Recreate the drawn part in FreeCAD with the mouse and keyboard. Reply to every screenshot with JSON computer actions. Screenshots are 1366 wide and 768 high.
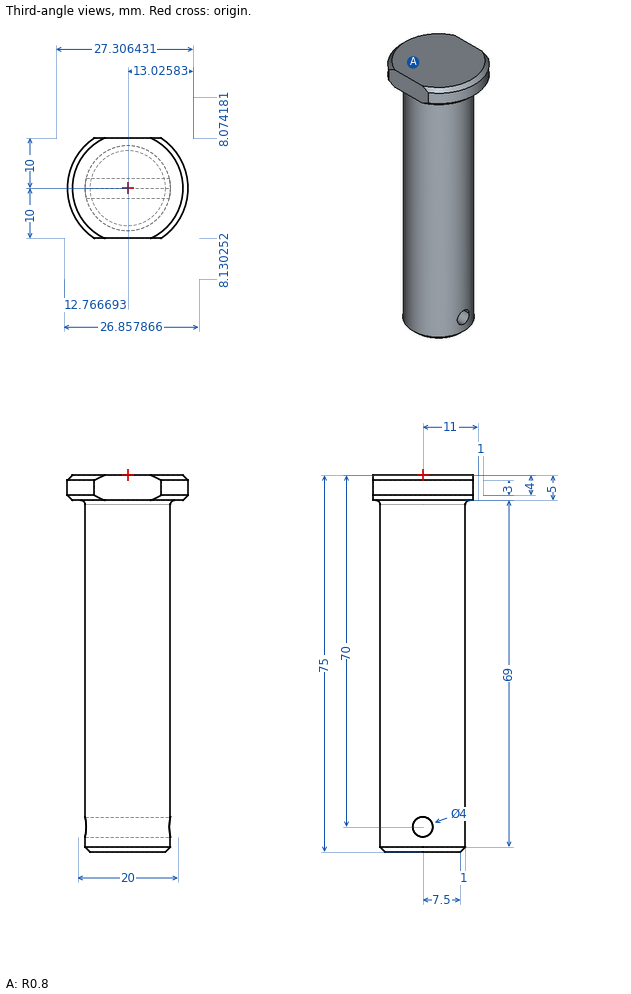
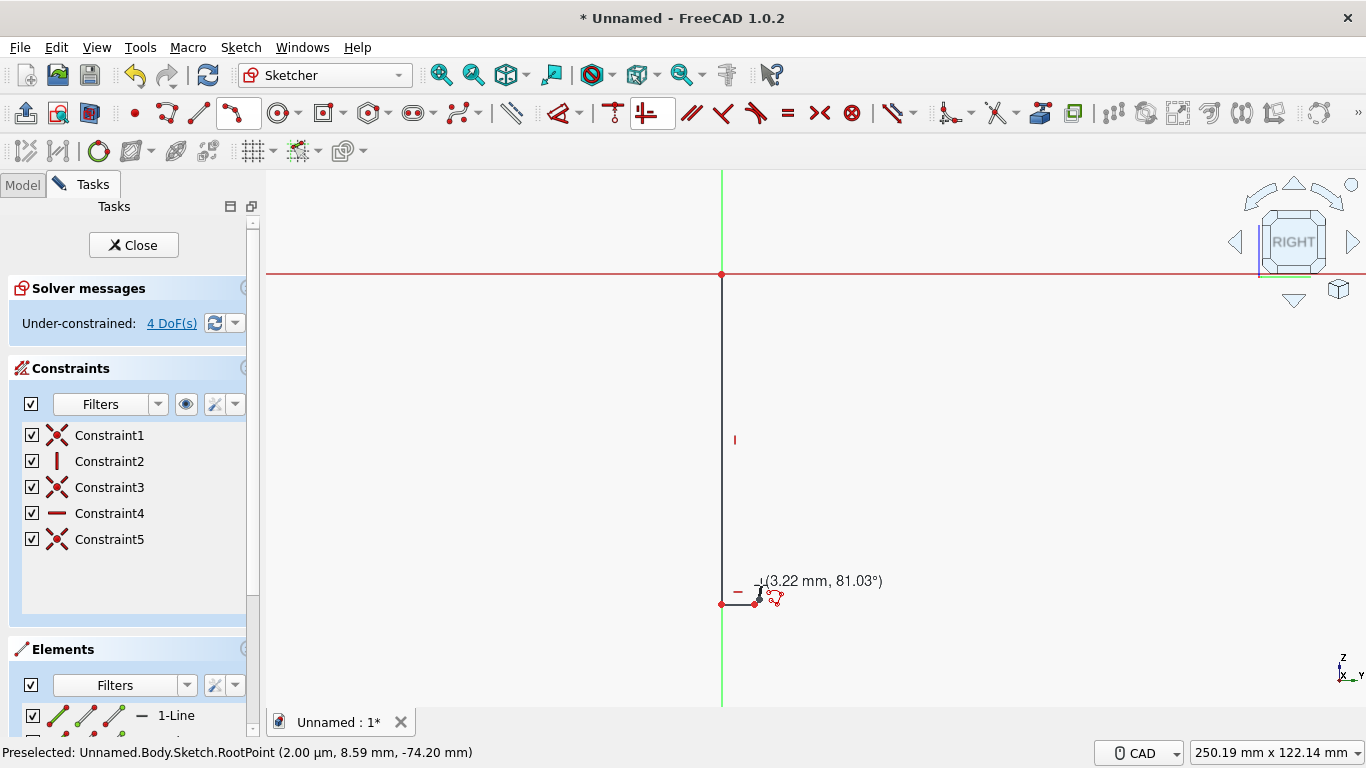
{"action": "left_click", "coordinate": [759, 296]}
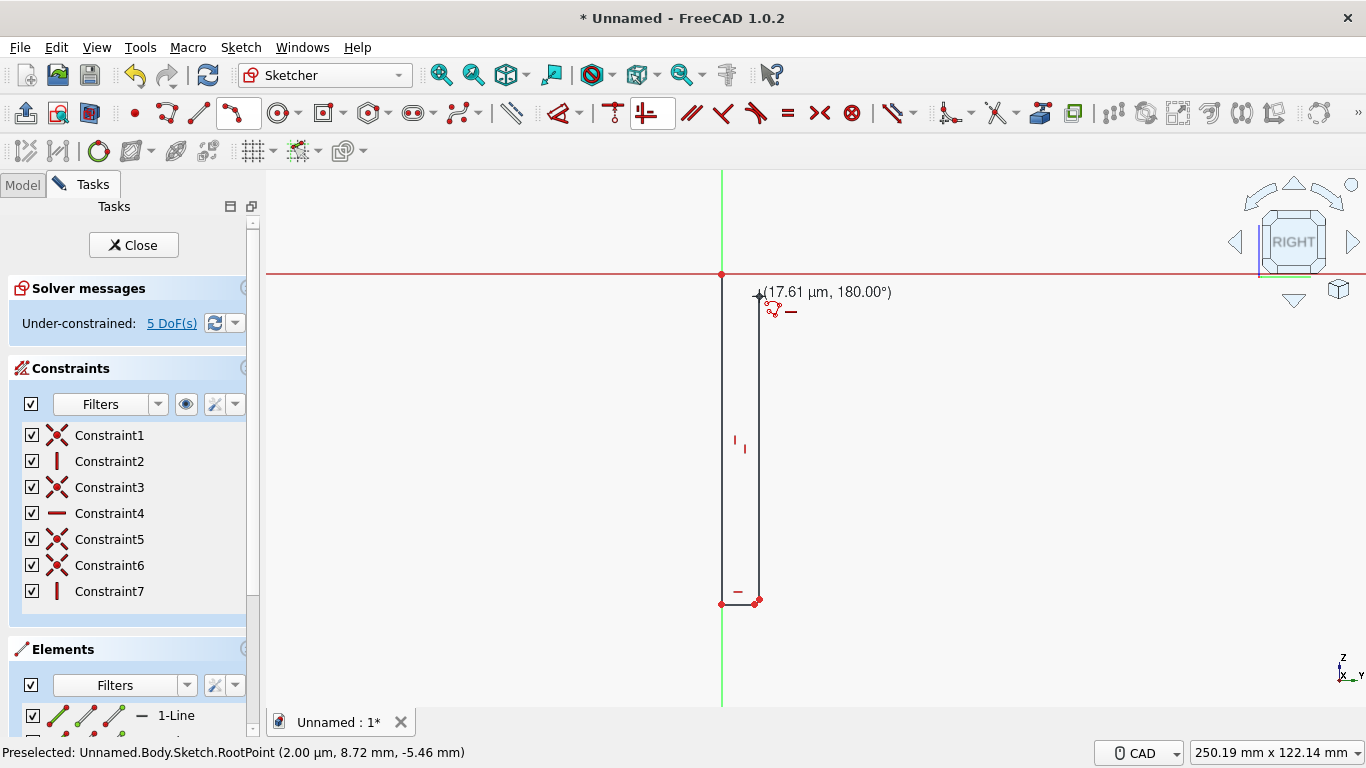
{"action": "scroll", "coordinate": [770, 296], "scroll_direction": "up", "scroll_amount": 2}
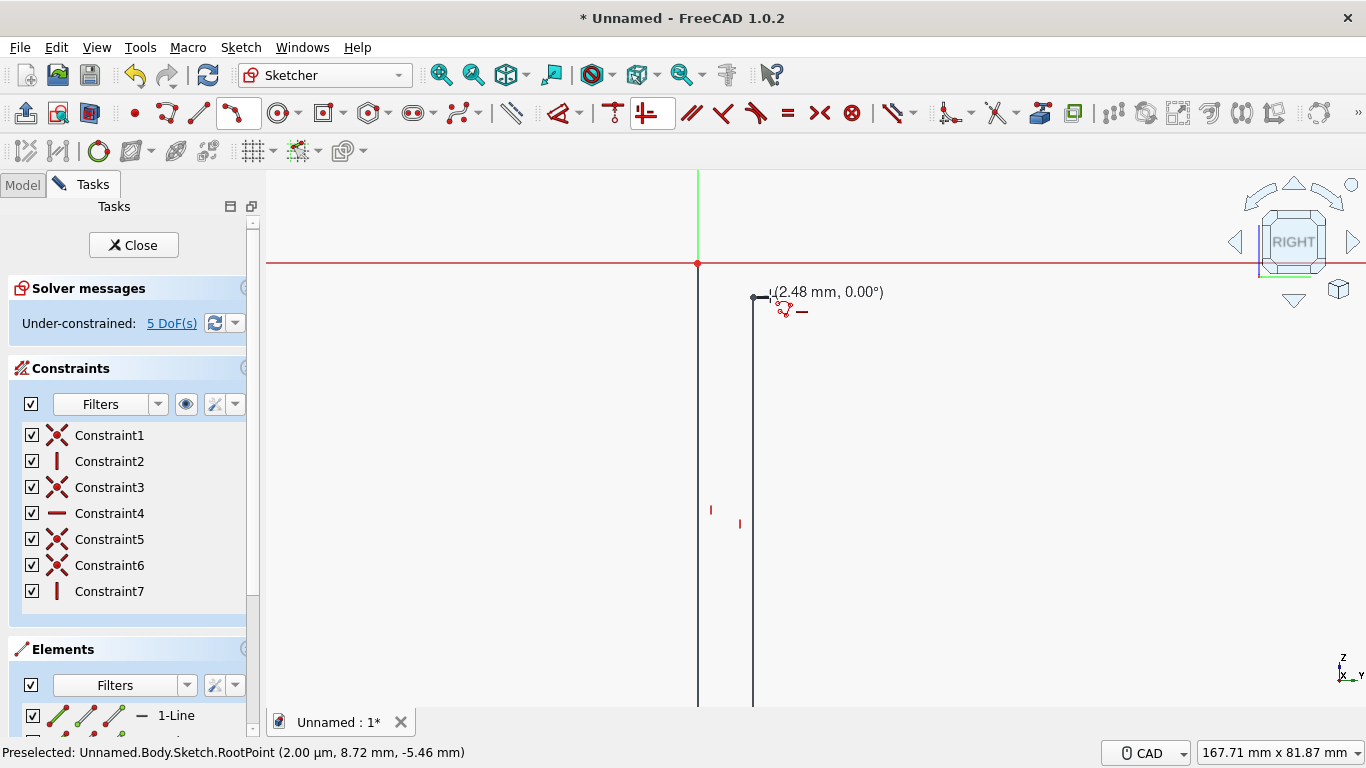
{"action": "left_click", "coordinate": [770, 296]}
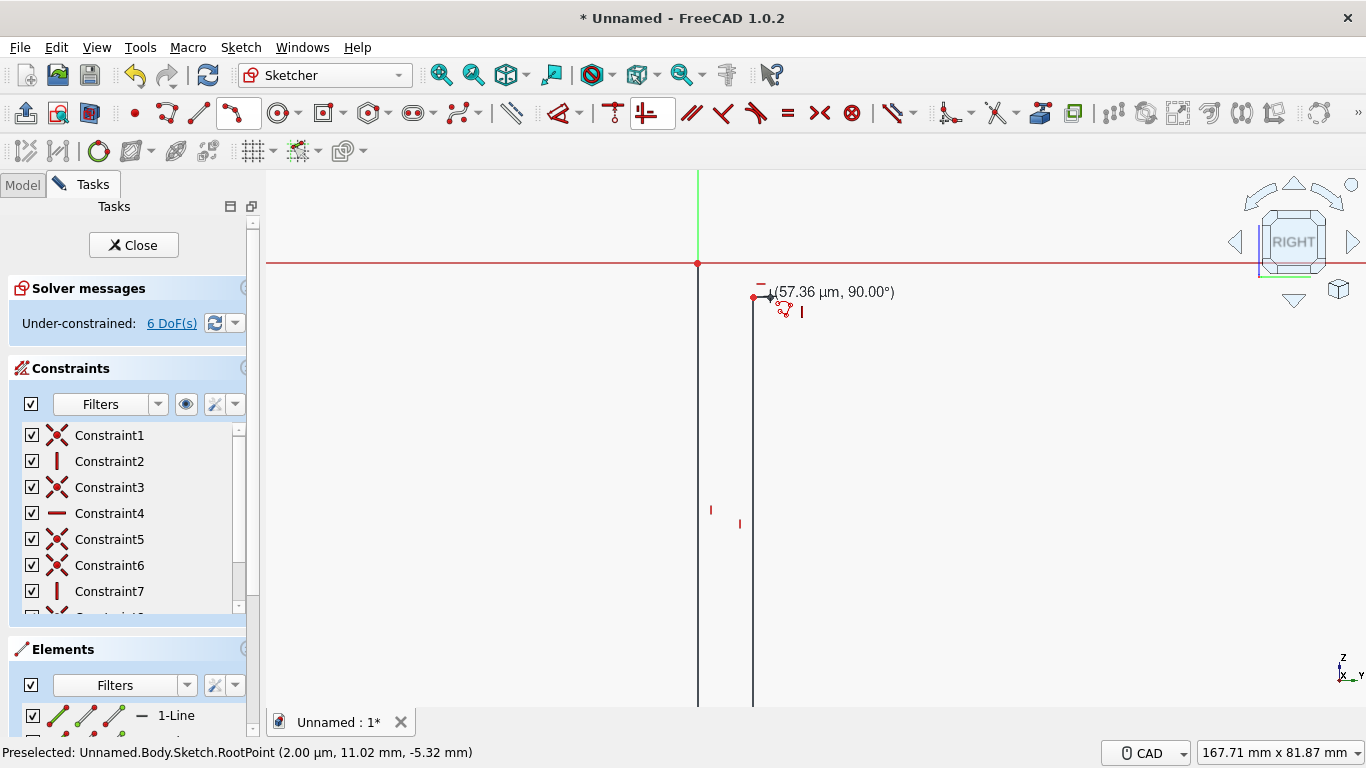
{"action": "scroll", "coordinate": [776, 289], "scroll_direction": "up", "scroll_amount": 3}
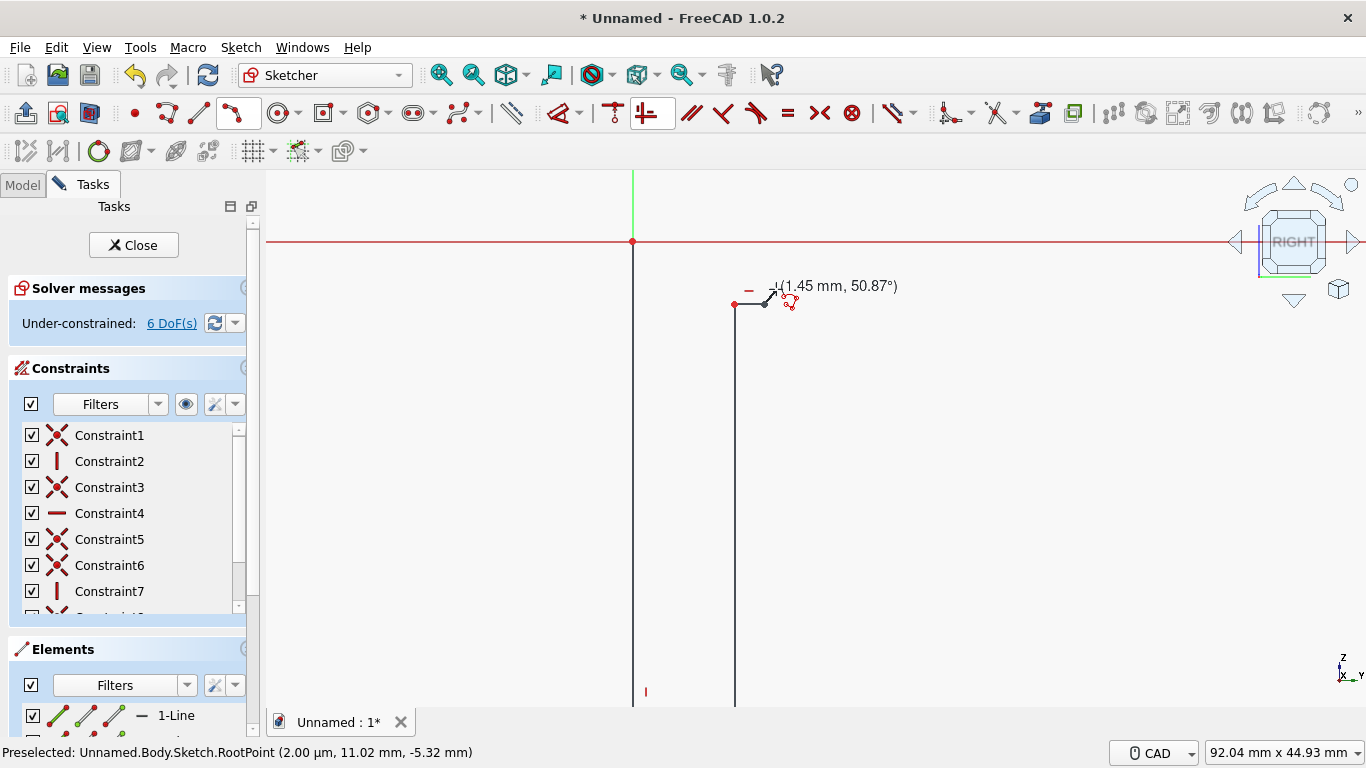
{"action": "left_click", "coordinate": [776, 289]}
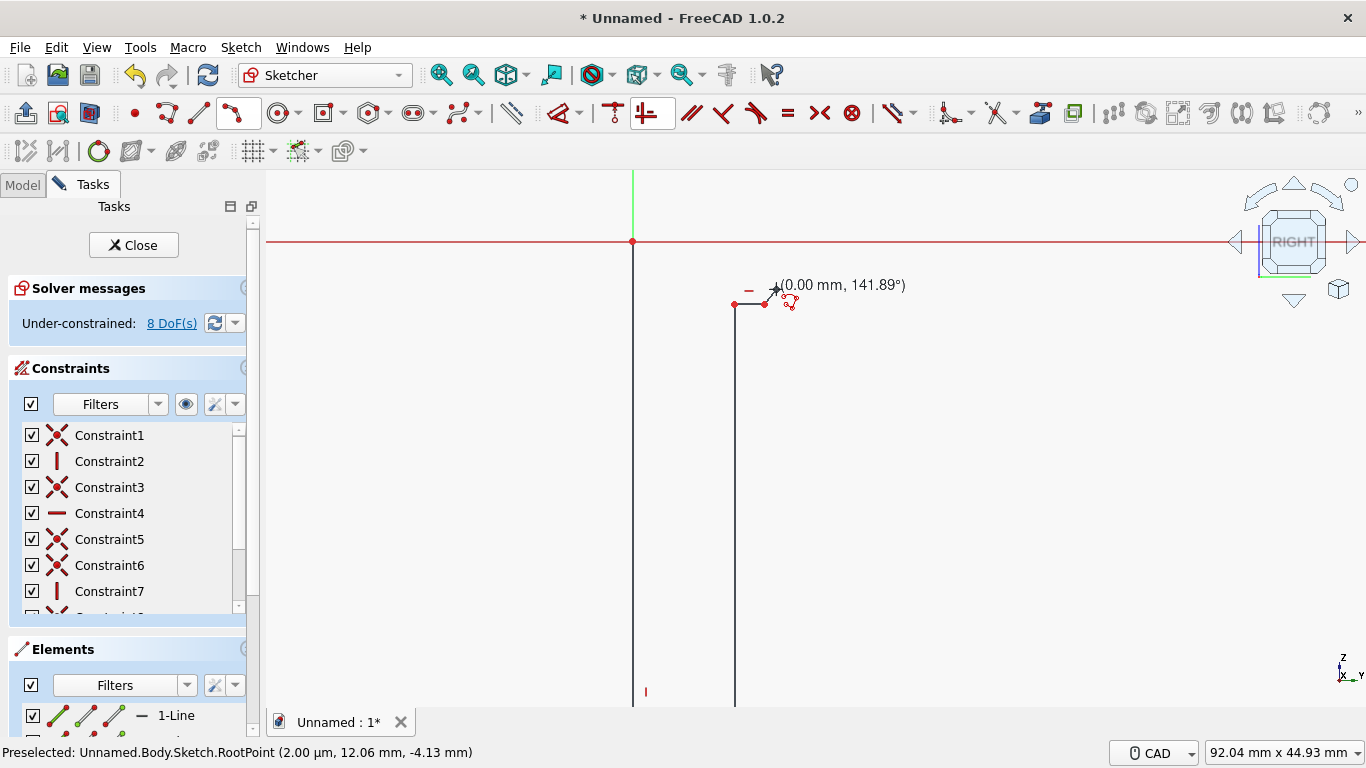
{"action": "scroll", "coordinate": [776, 254], "scroll_direction": "up", "scroll_amount": 2}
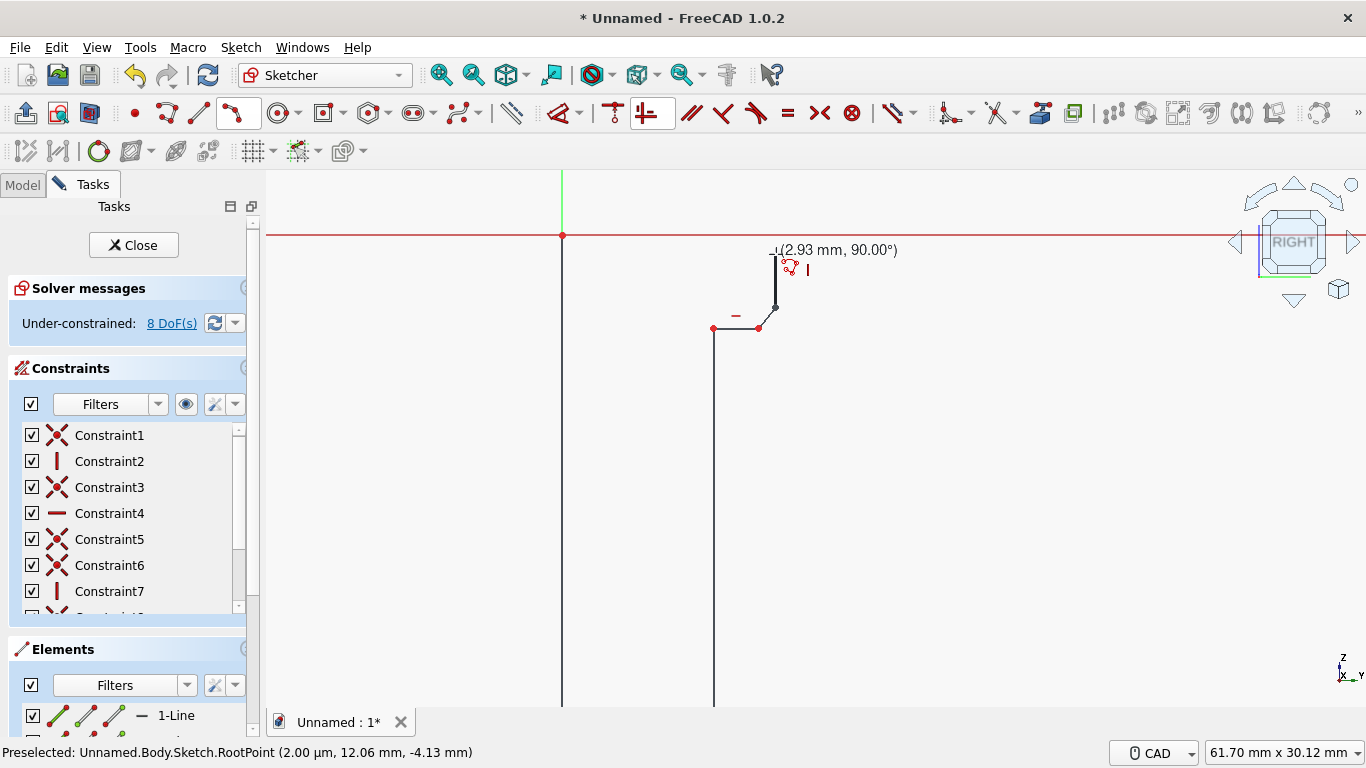
{"action": "left_click", "coordinate": [776, 253]}
{"action": "left_click", "coordinate": [758, 244]}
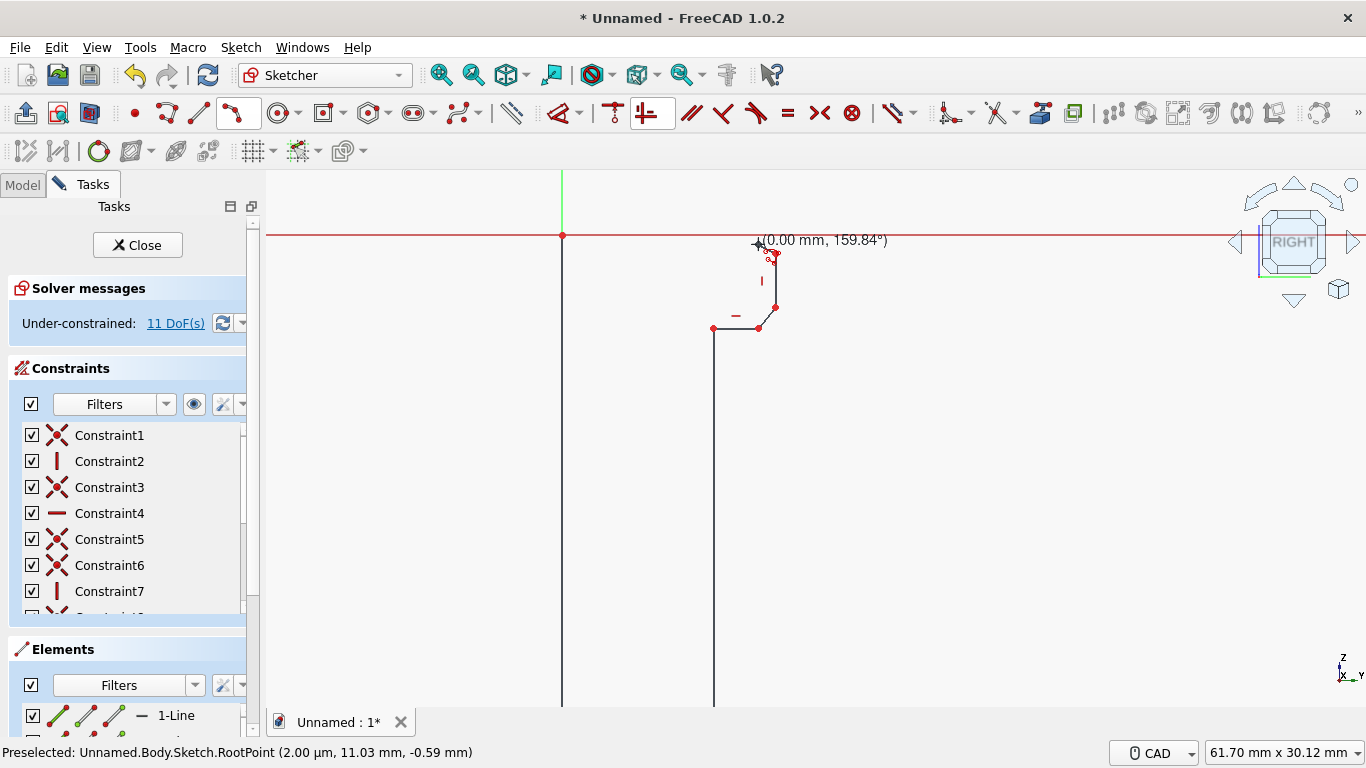
{"action": "scroll", "coordinate": [773, 286], "scroll_direction": "down", "scroll_amount": 7}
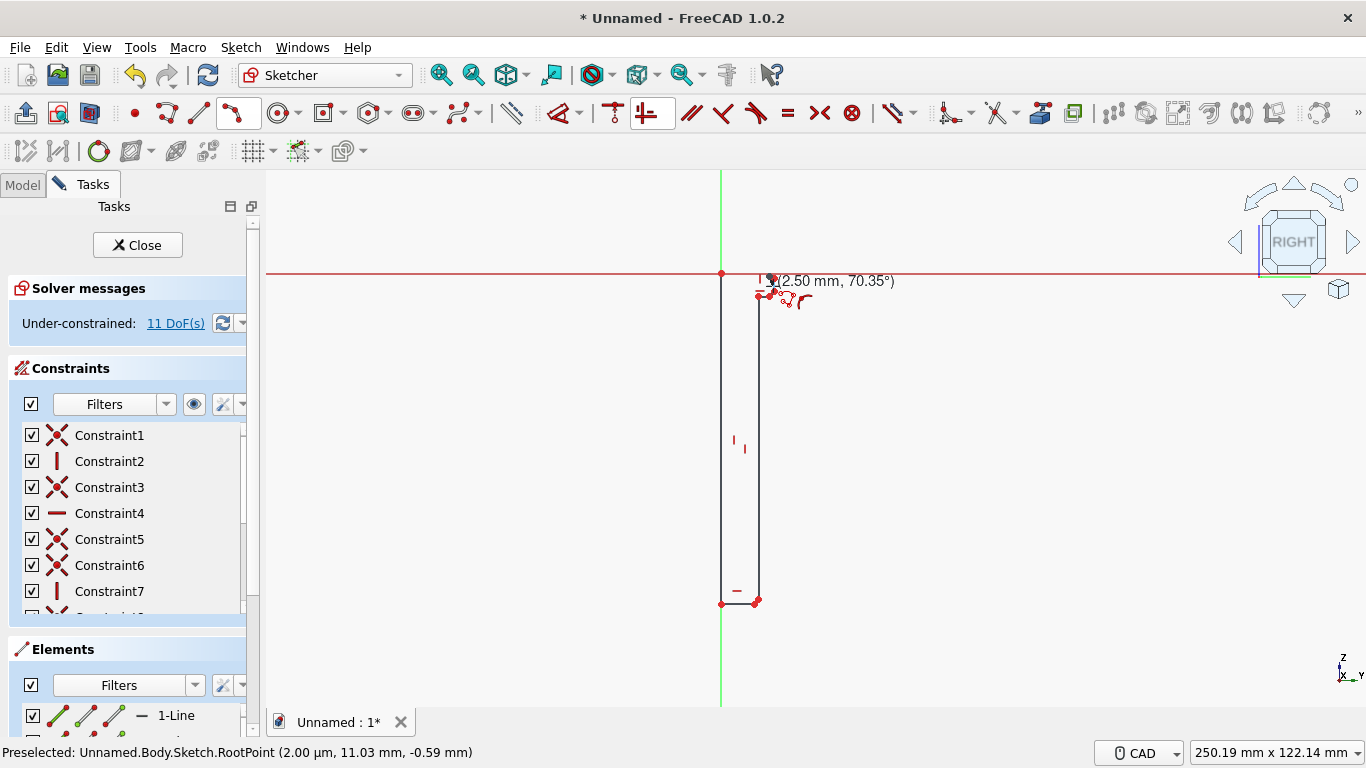
{"action": "left_click", "coordinate": [721, 274]}
{"action": "key", "text": "Escape"}
{"action": "key", "text": "Escape"}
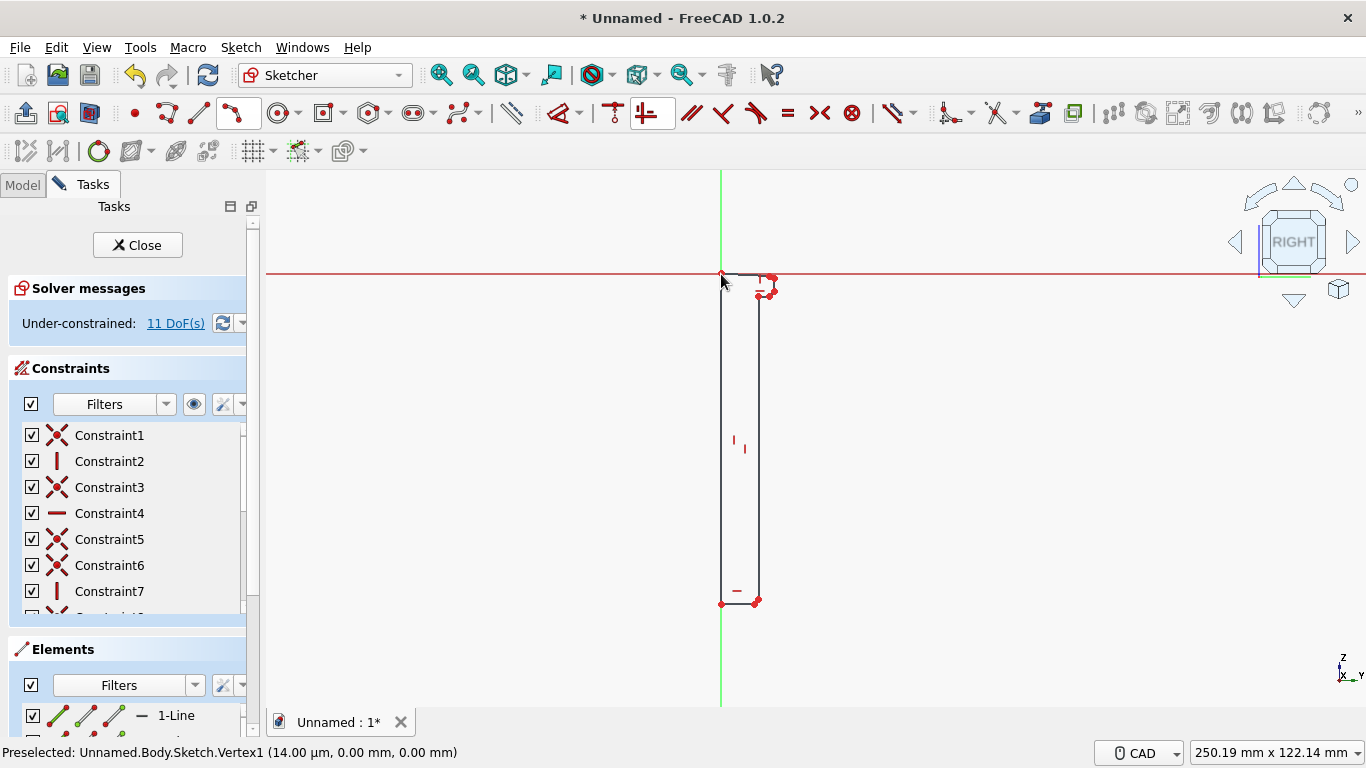
{"action": "left_click", "coordinate": [736, 274]}